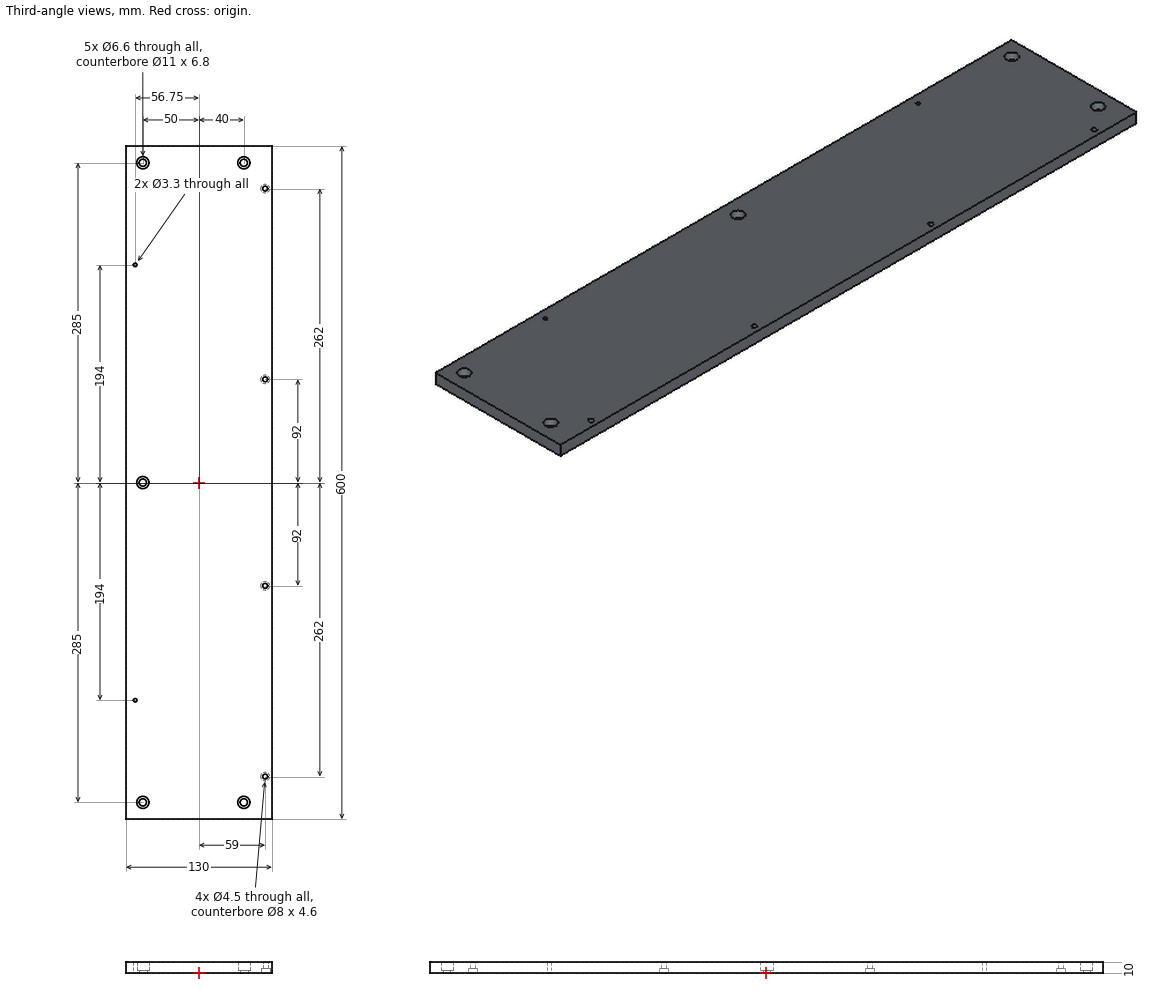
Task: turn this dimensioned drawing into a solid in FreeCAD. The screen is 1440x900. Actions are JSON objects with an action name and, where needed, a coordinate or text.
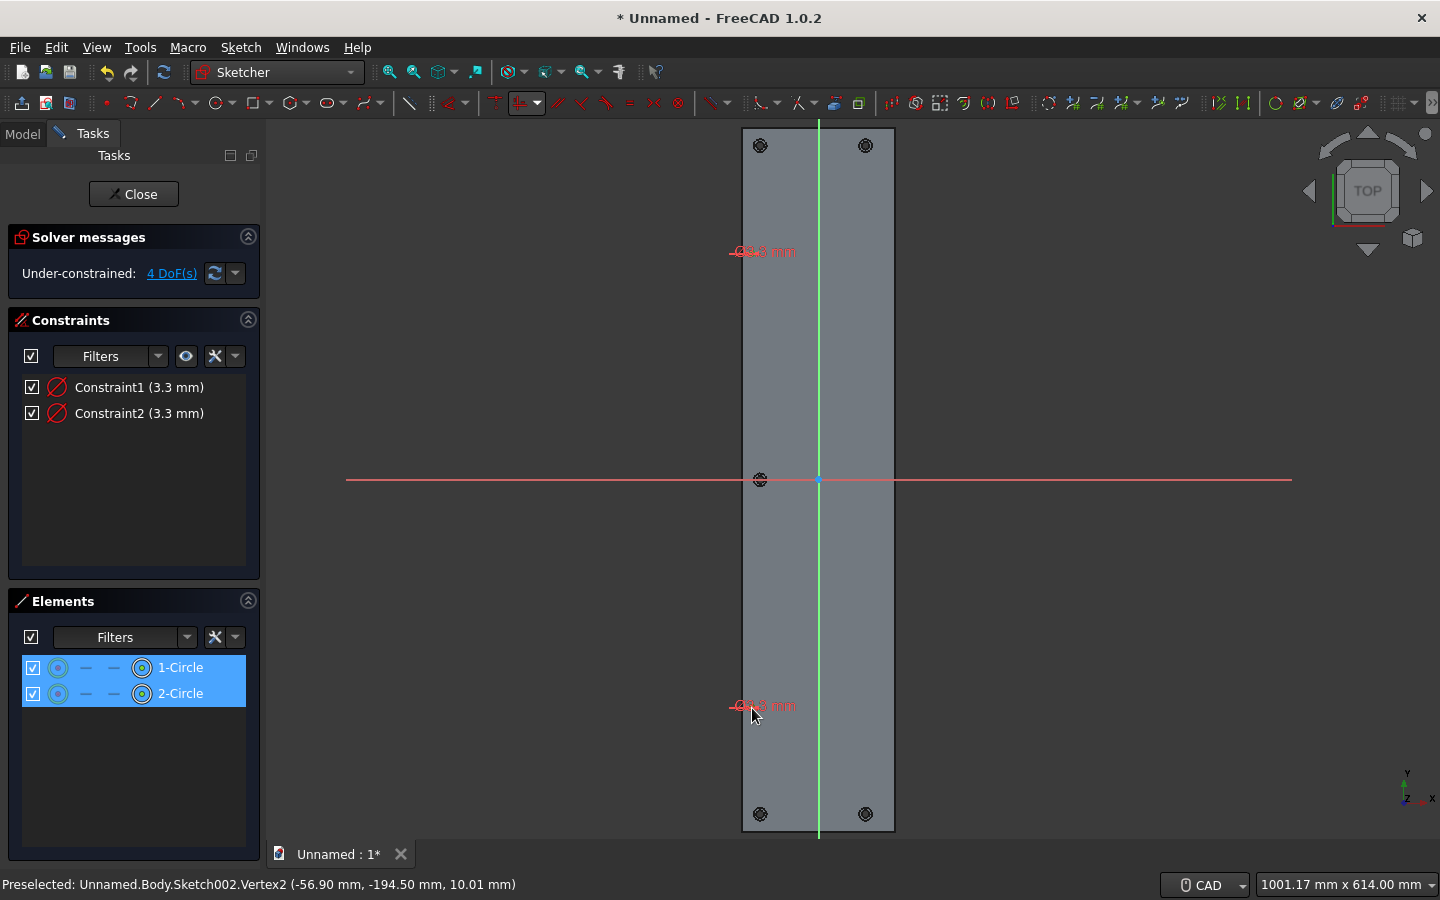
{"action": "key", "text": "v"}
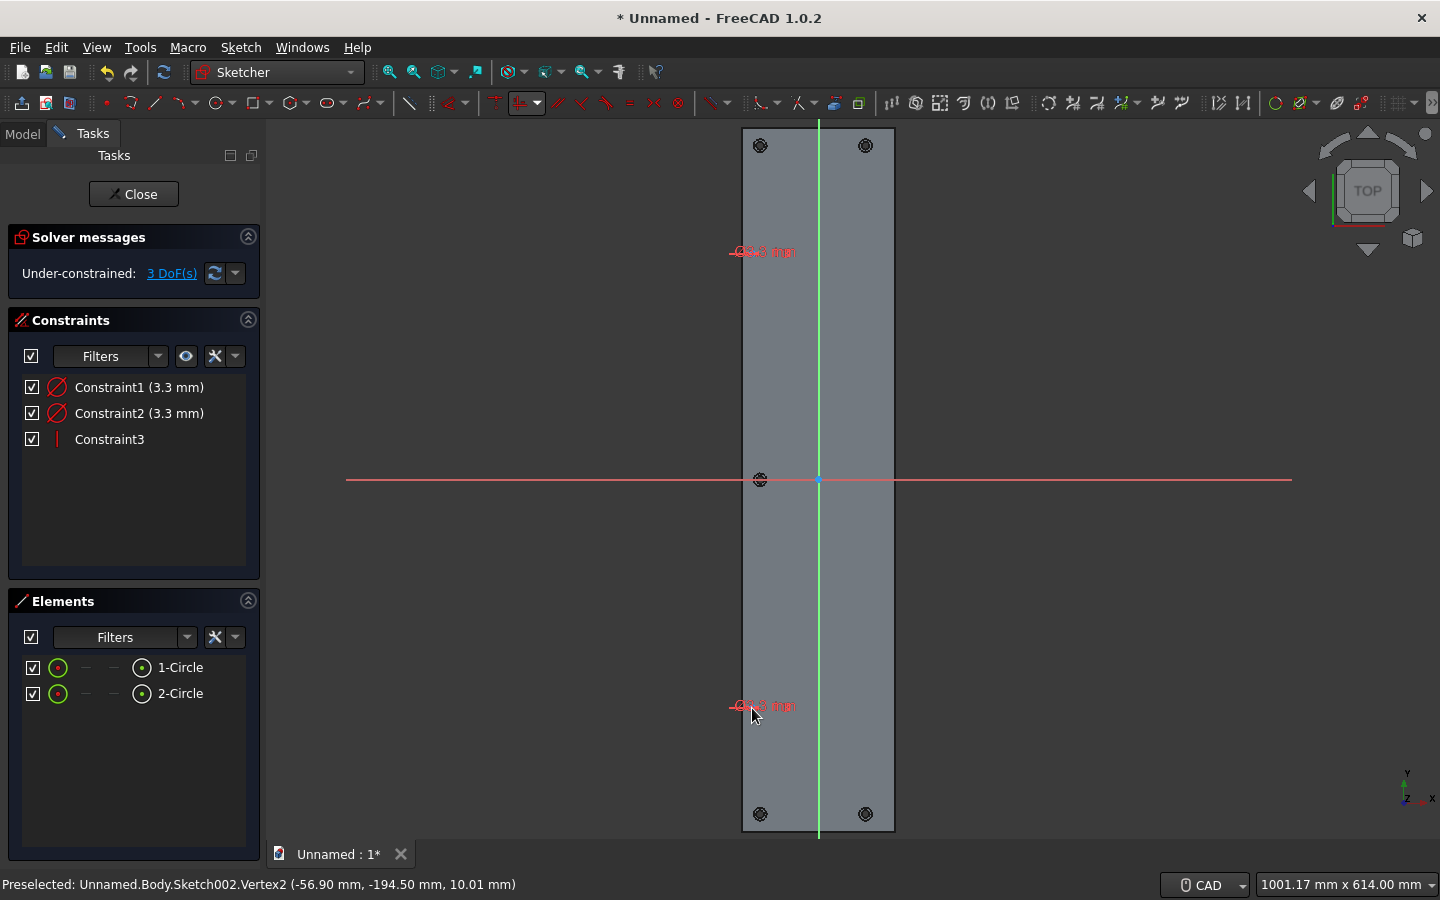
{"action": "left_click", "coordinate": [448, 104]}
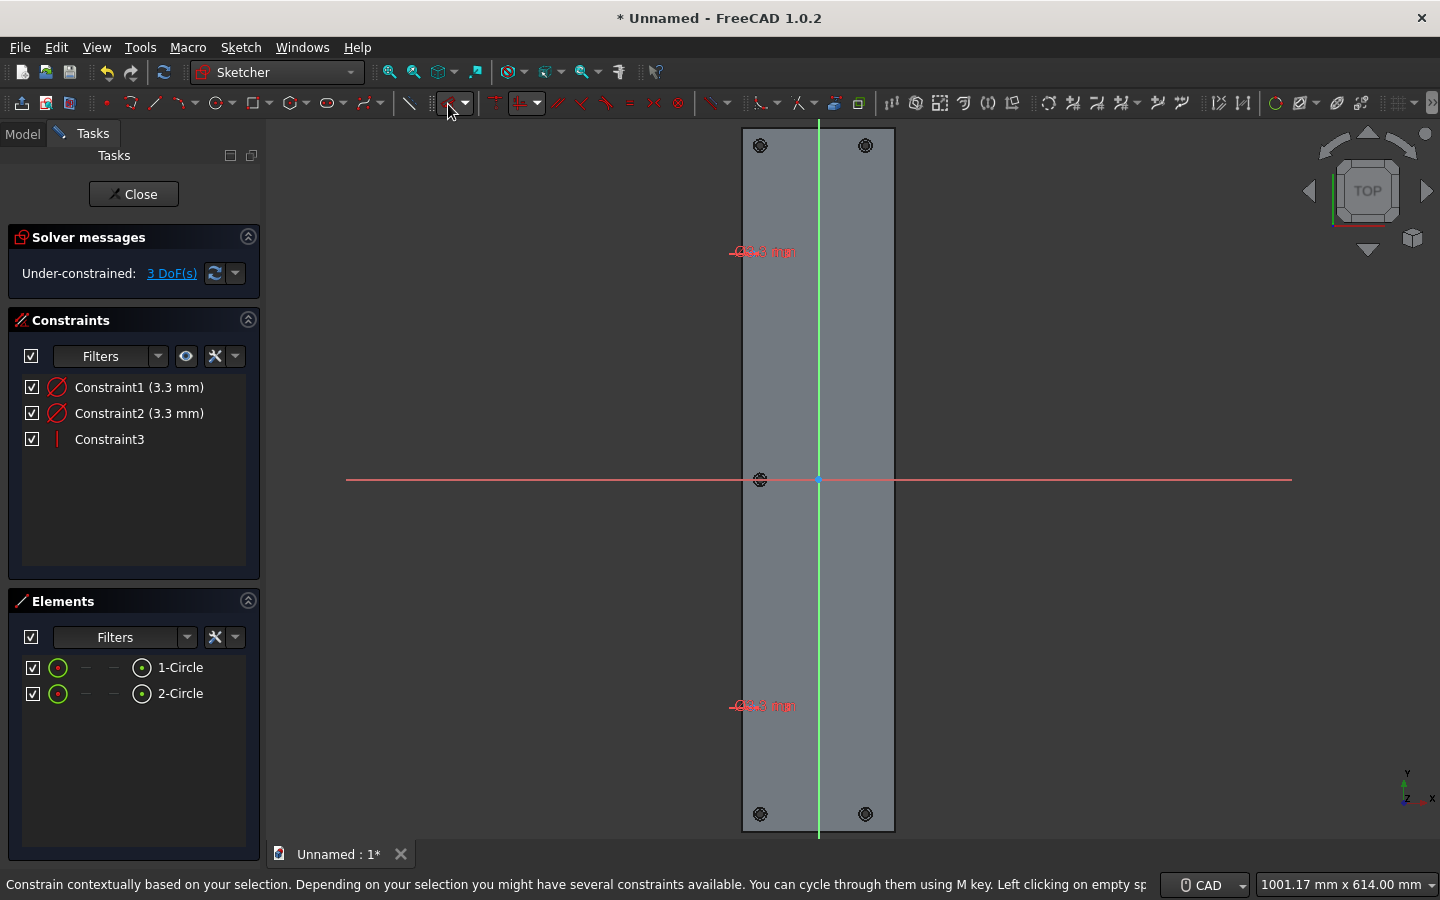
{"action": "left_click", "coordinate": [752, 254]}
{"action": "left_click", "coordinate": [853, 367]}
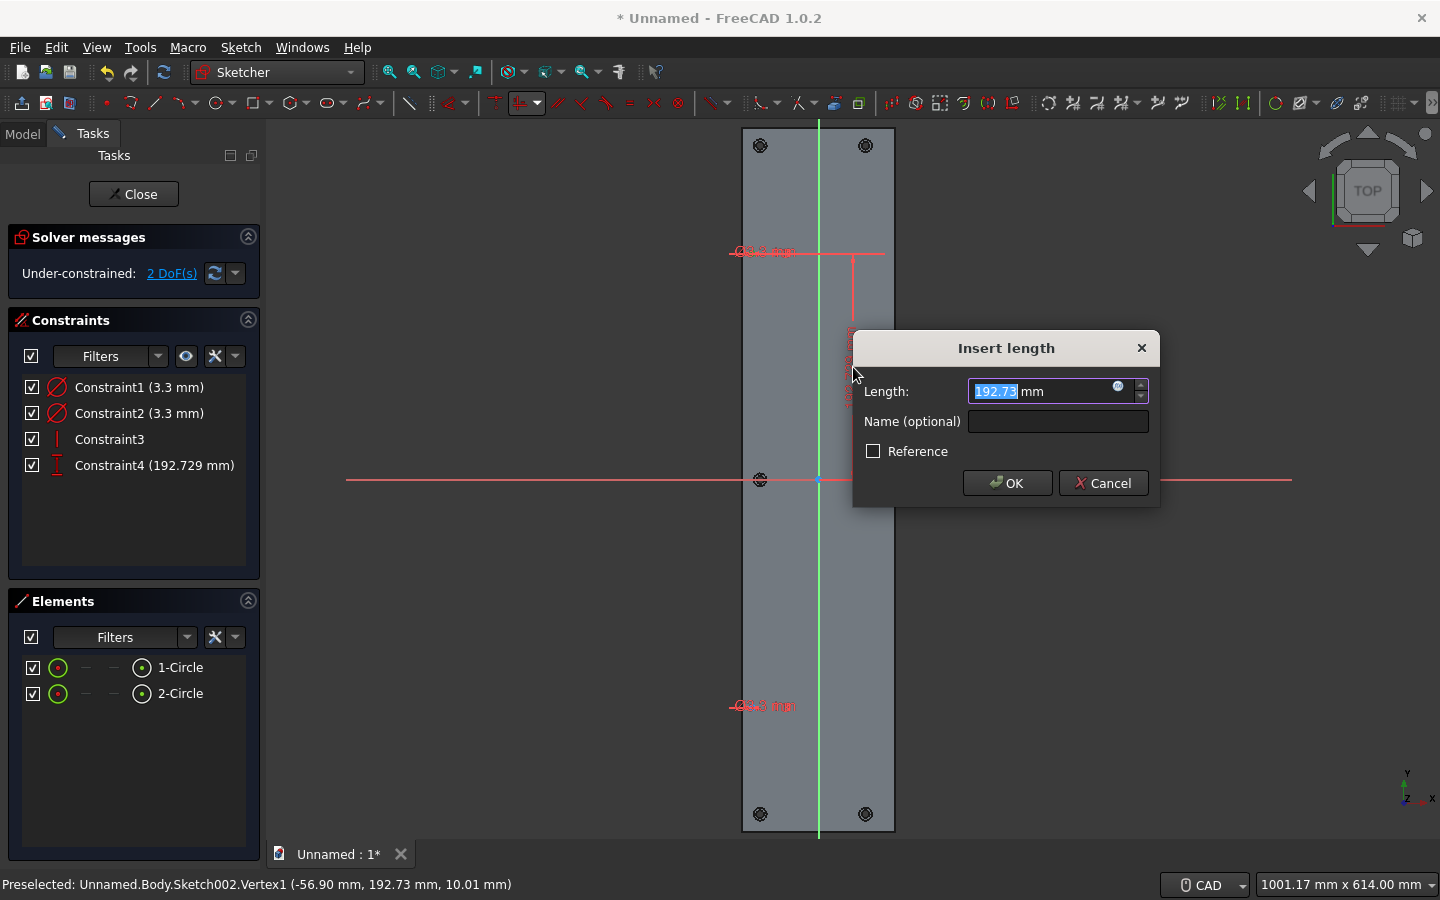
{"action": "type", "text": "194"}
{"action": "key", "text": "Return"}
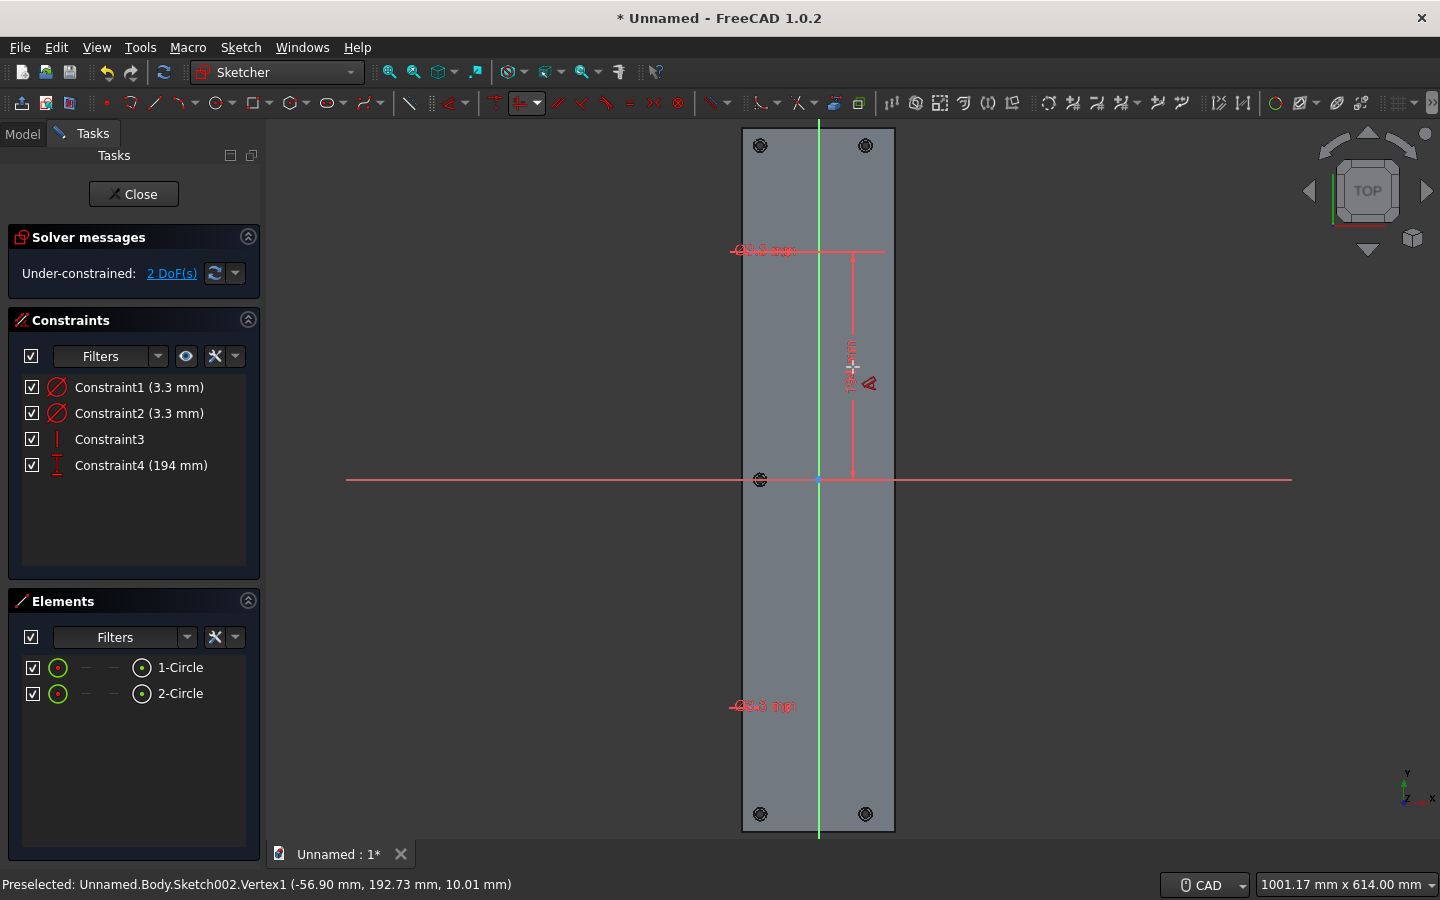
{"action": "left_click", "coordinate": [752, 708]}
{"action": "left_click", "coordinate": [853, 594]}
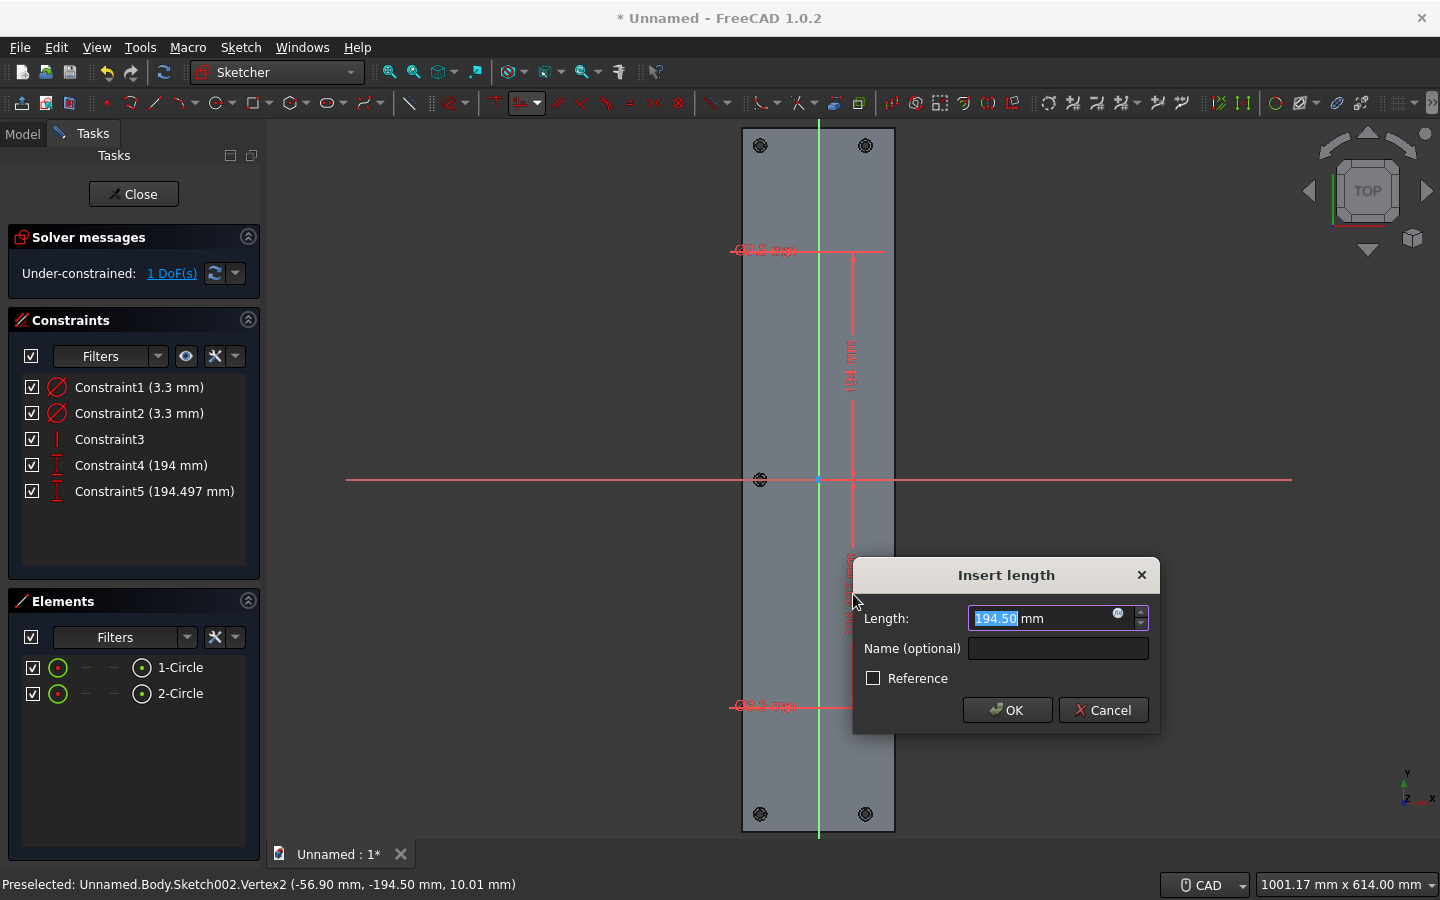
{"action": "type", "text": "194"}
{"action": "key", "text": "Return"}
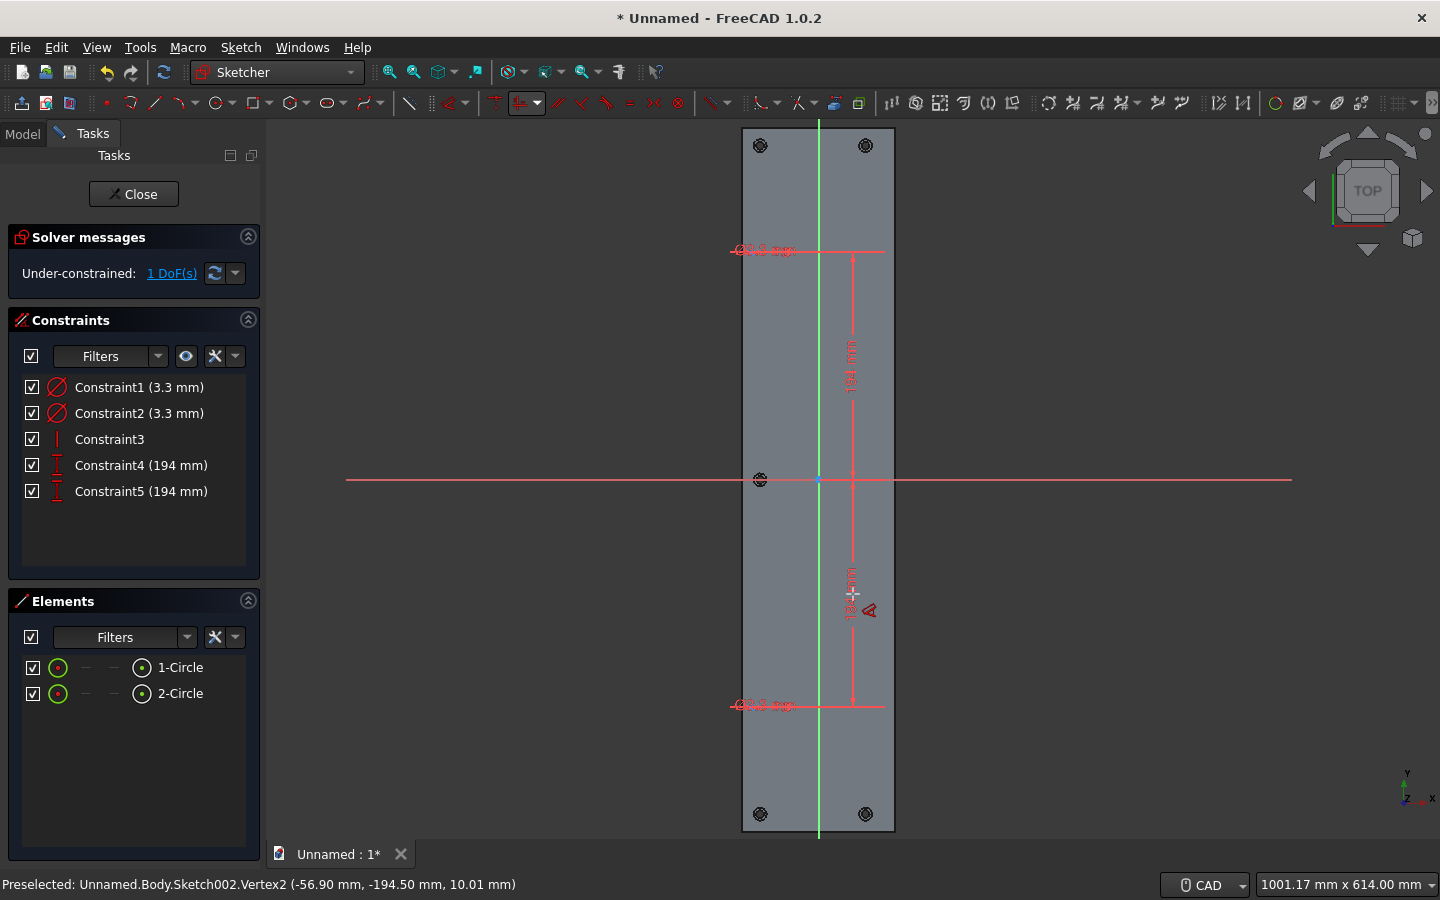
{"action": "left_click", "coordinate": [752, 252]}
{"action": "left_click", "coordinate": [785, 218]}